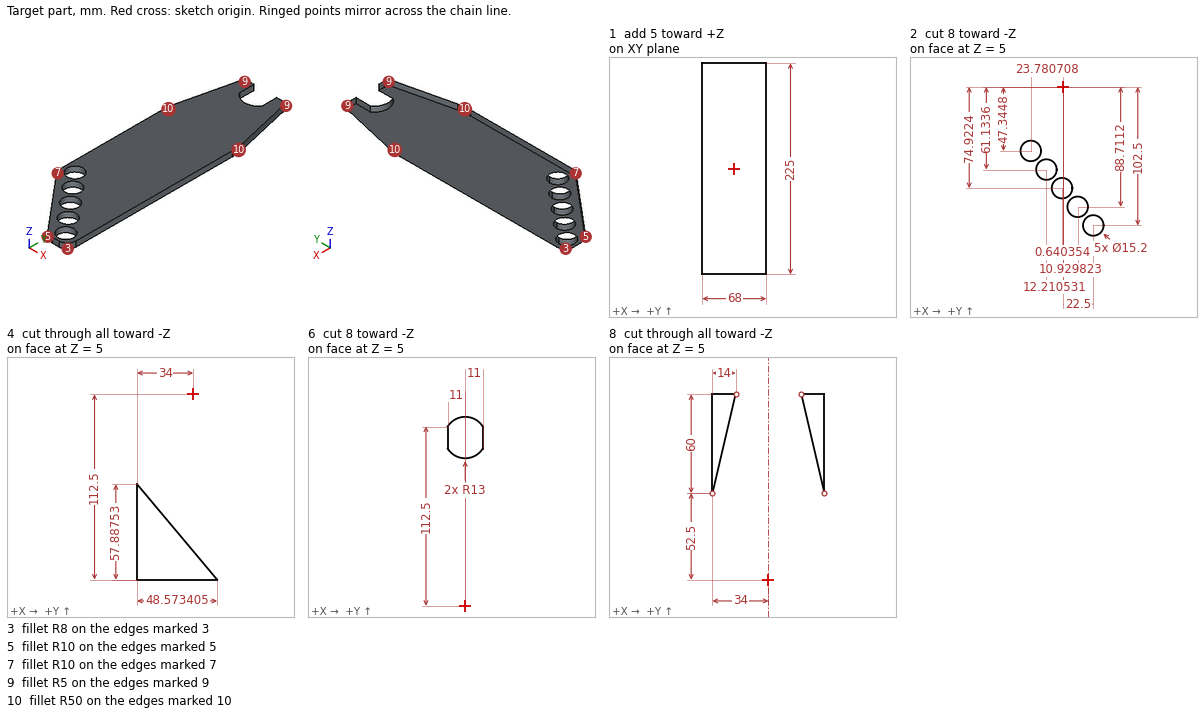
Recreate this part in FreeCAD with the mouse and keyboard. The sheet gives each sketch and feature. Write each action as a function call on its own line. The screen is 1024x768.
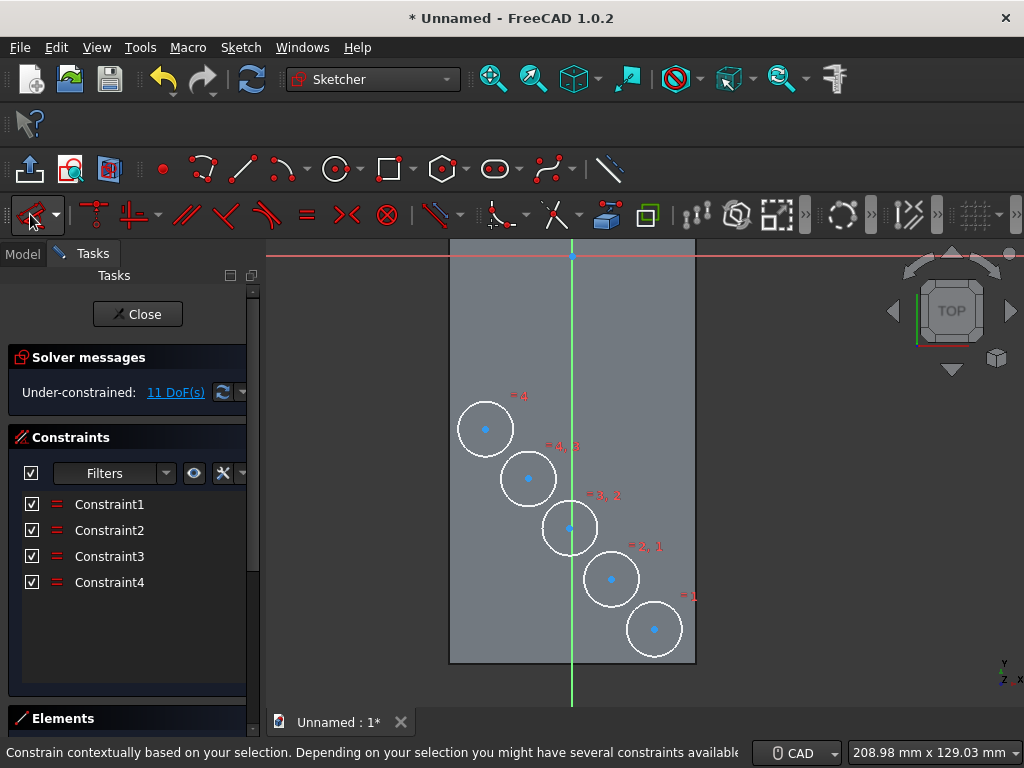
click(674, 610)
click(697, 588)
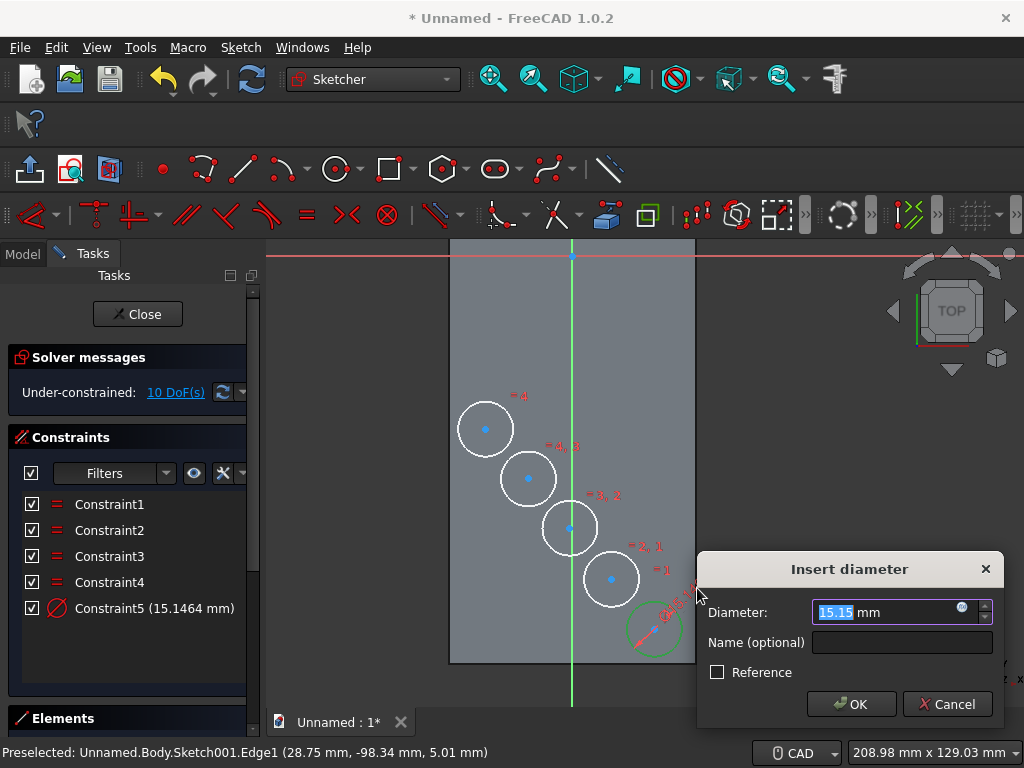
text(15.2)
key(Return)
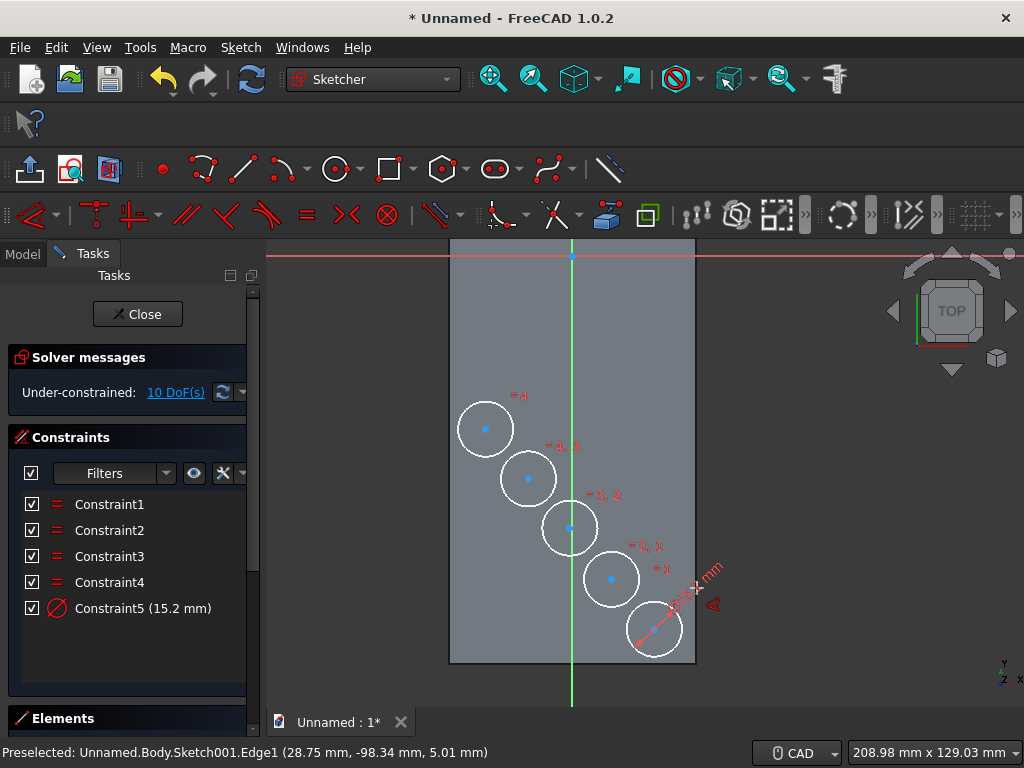
click(654, 629)
click(613, 663)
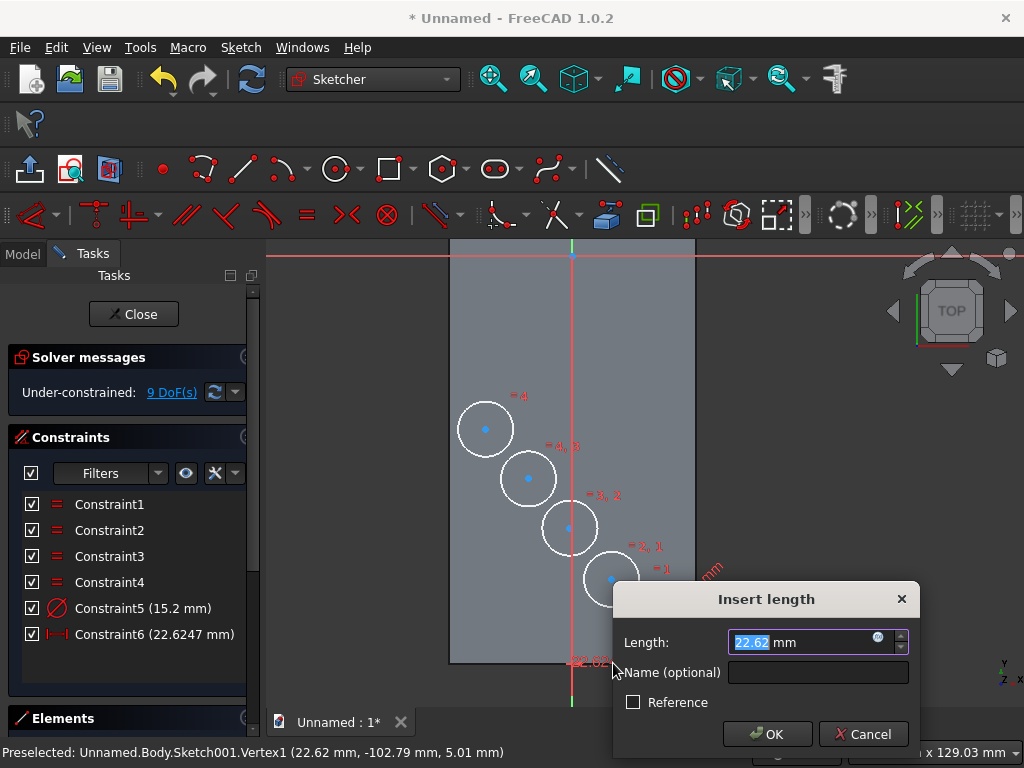
text(22.5)
key(Return)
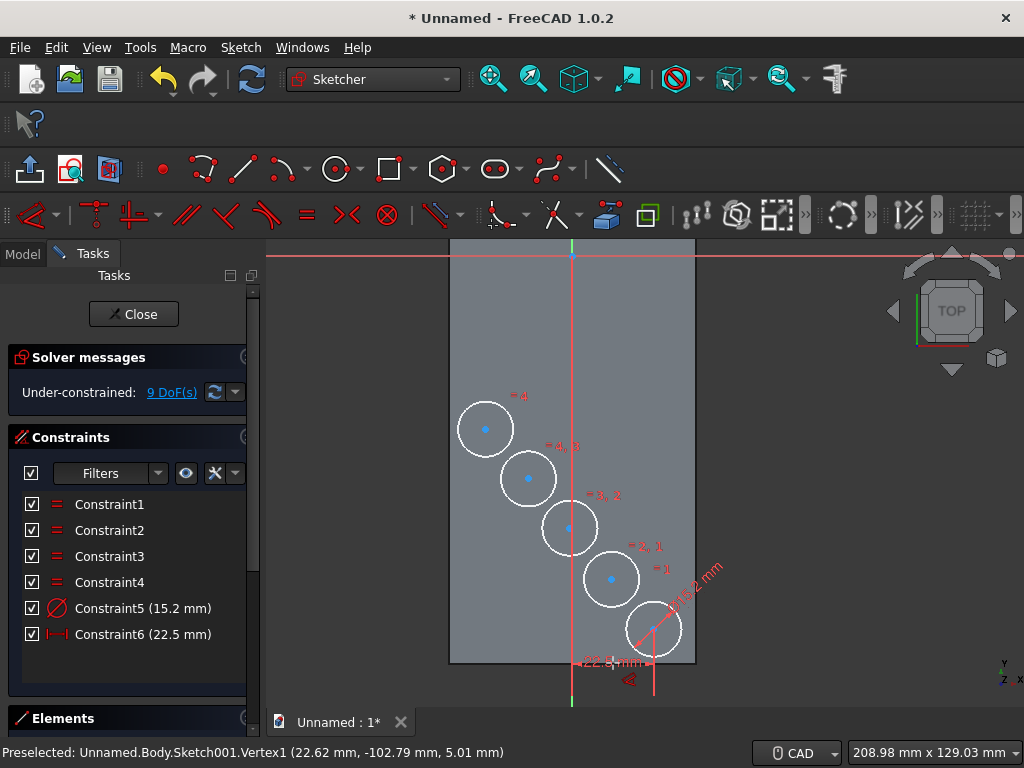
click(654, 629)
click(688, 448)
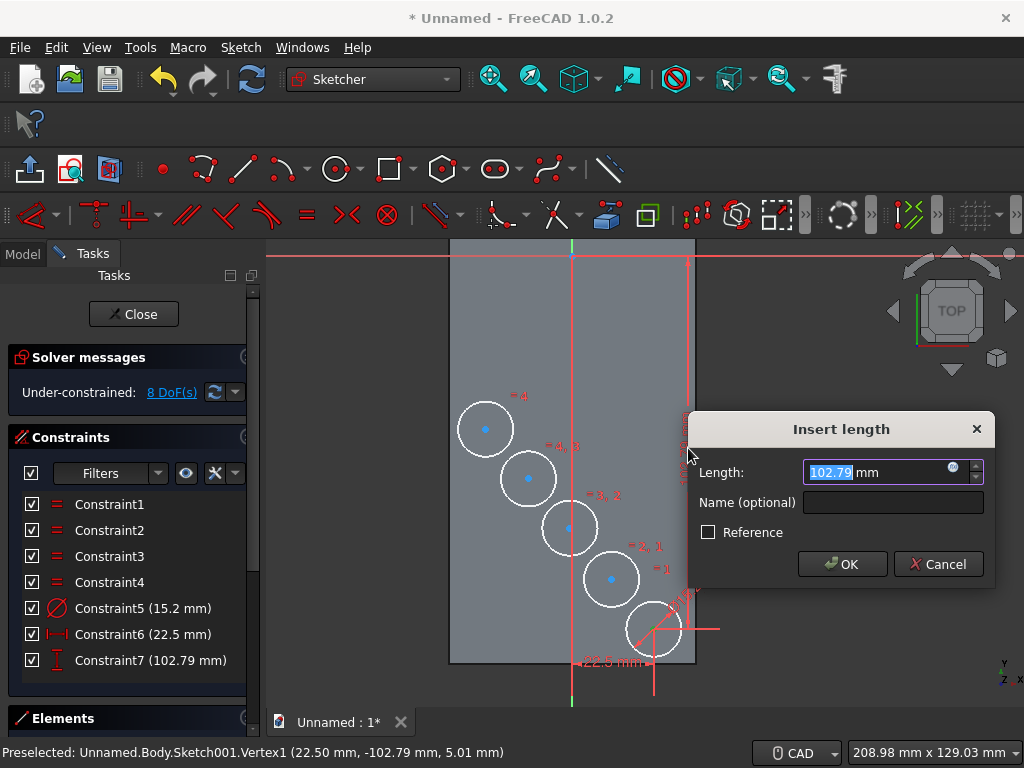
text(102.5)
key(Return)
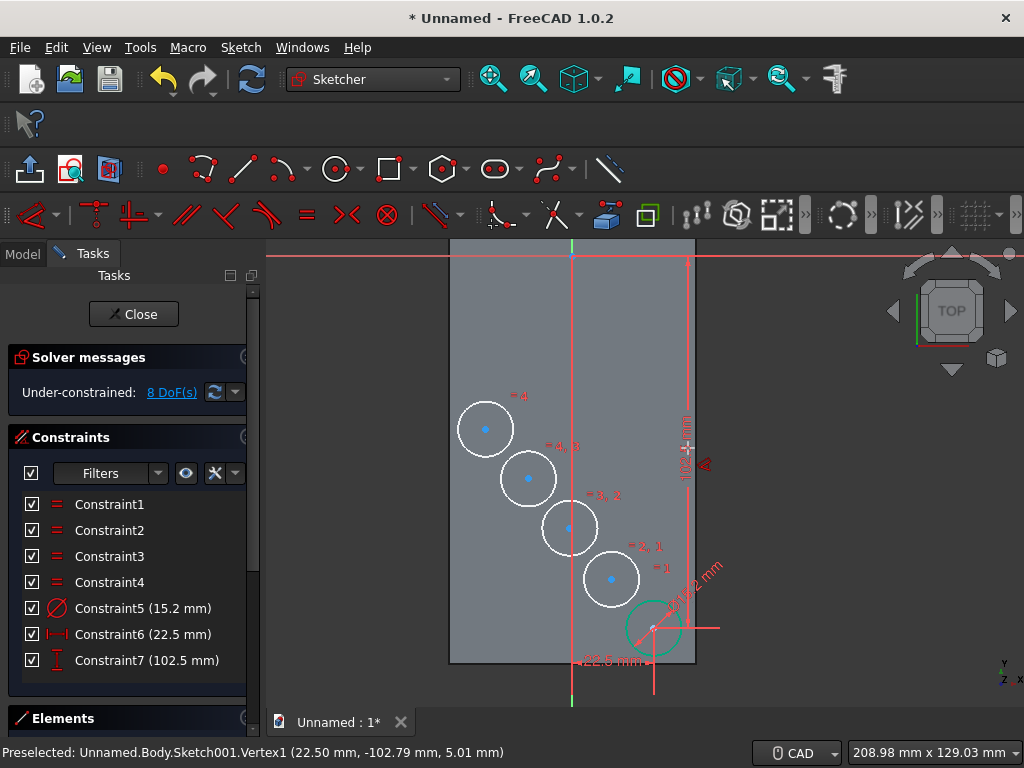
click(612, 579)
click(646, 423)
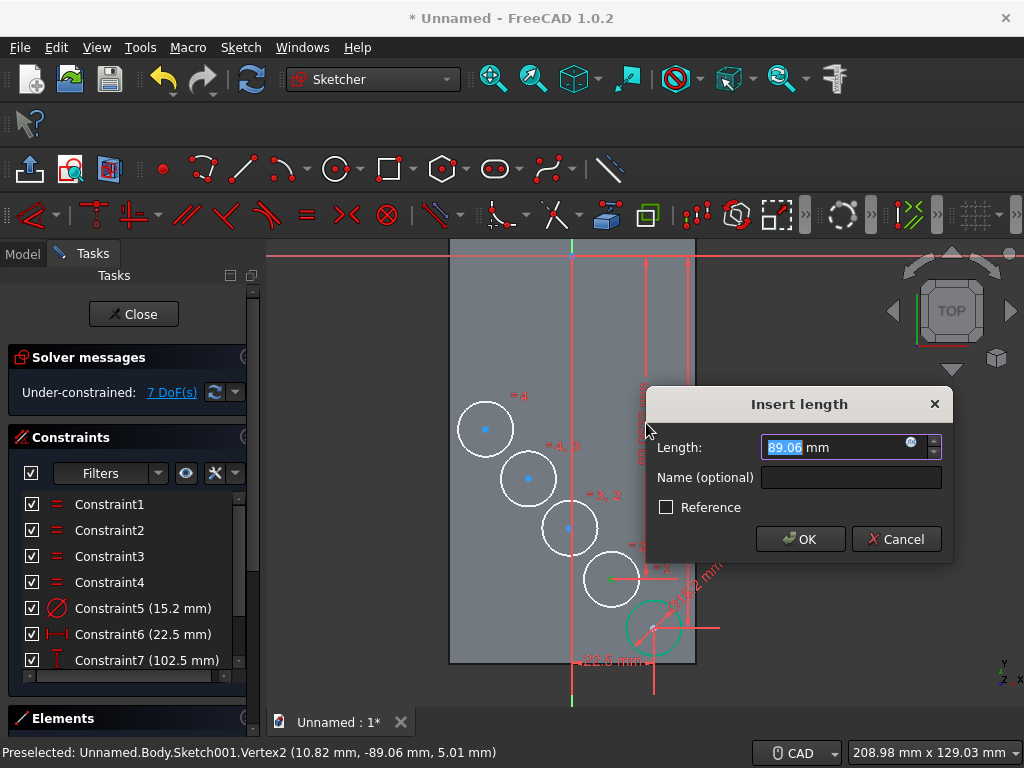
text(88.7112)
key(Return)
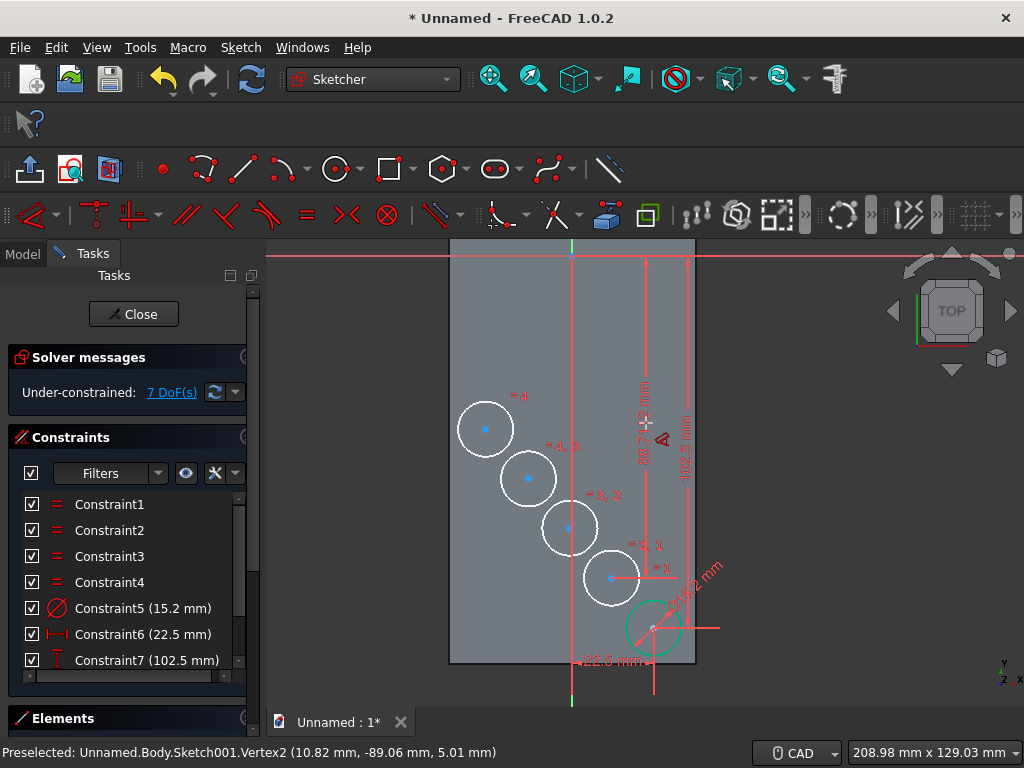
click(570, 528)
click(606, 398)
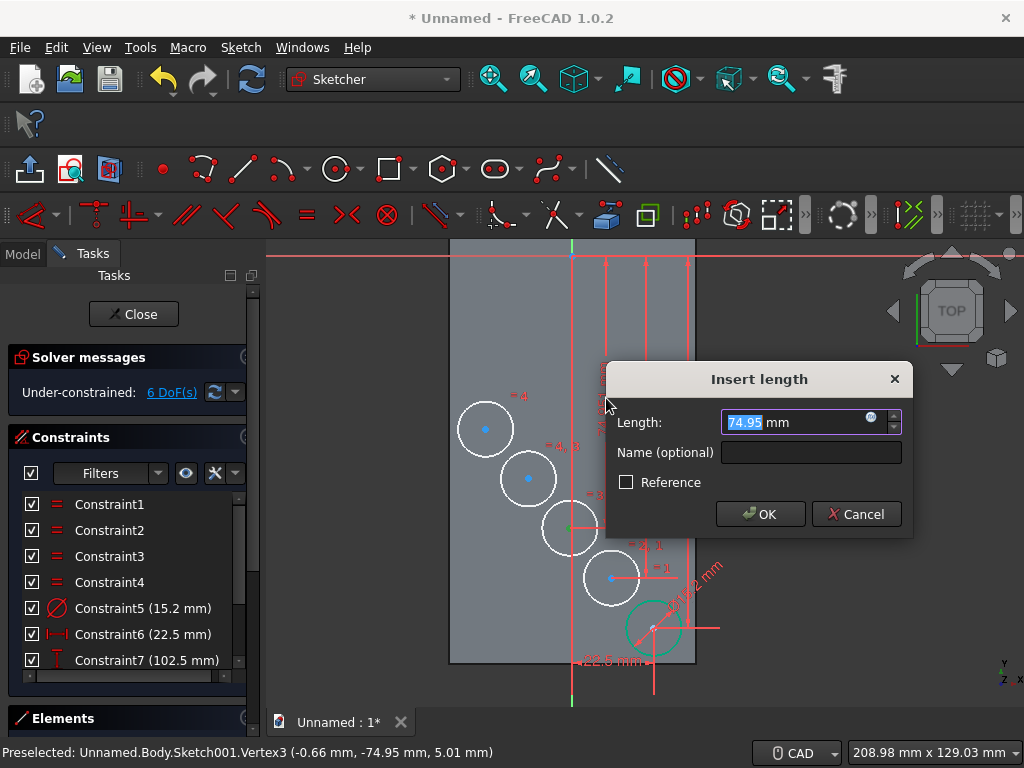
text(74.9224)
key(Return)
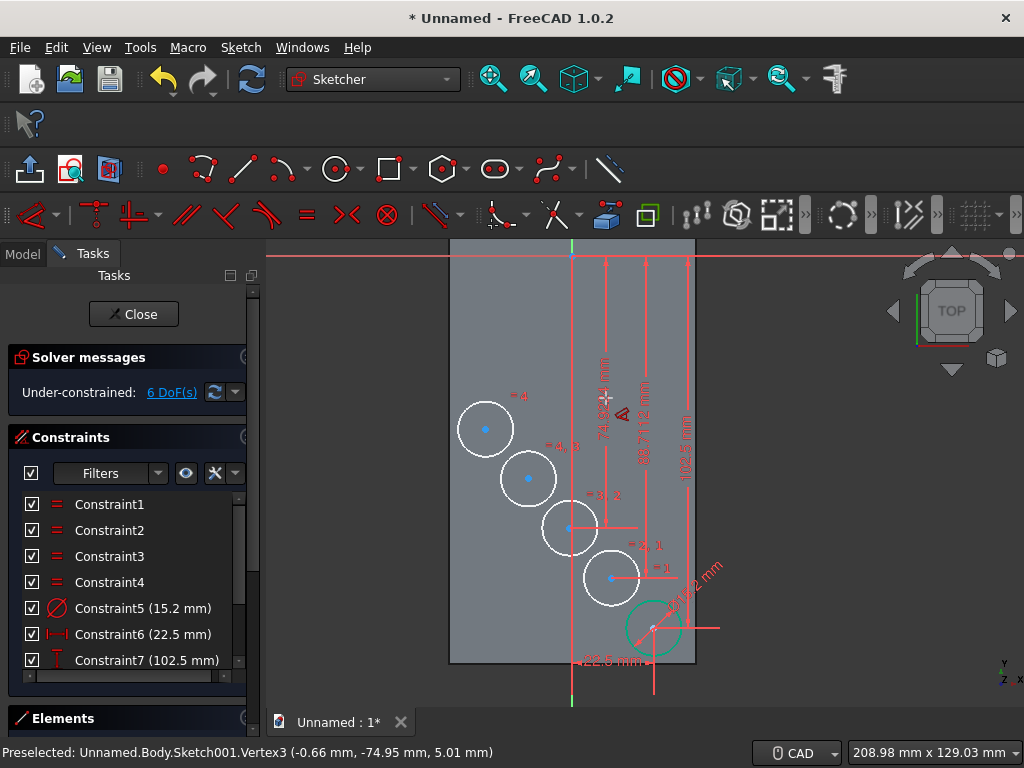
click(528, 479)
click(494, 373)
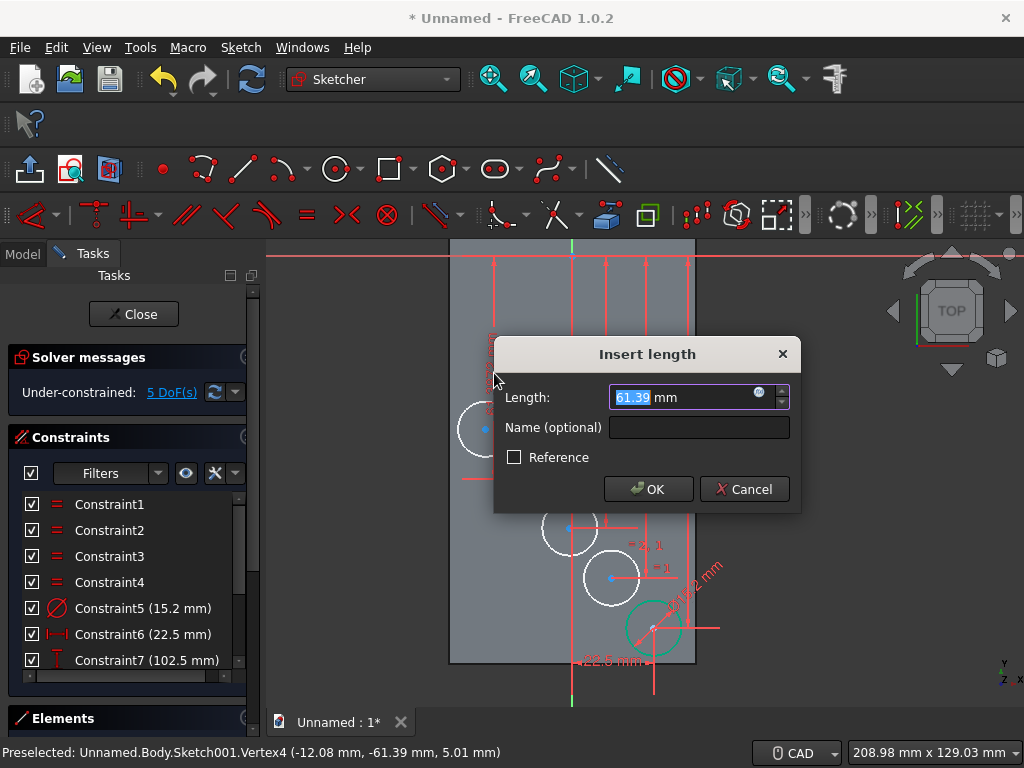
text(61.1336)
key(Return)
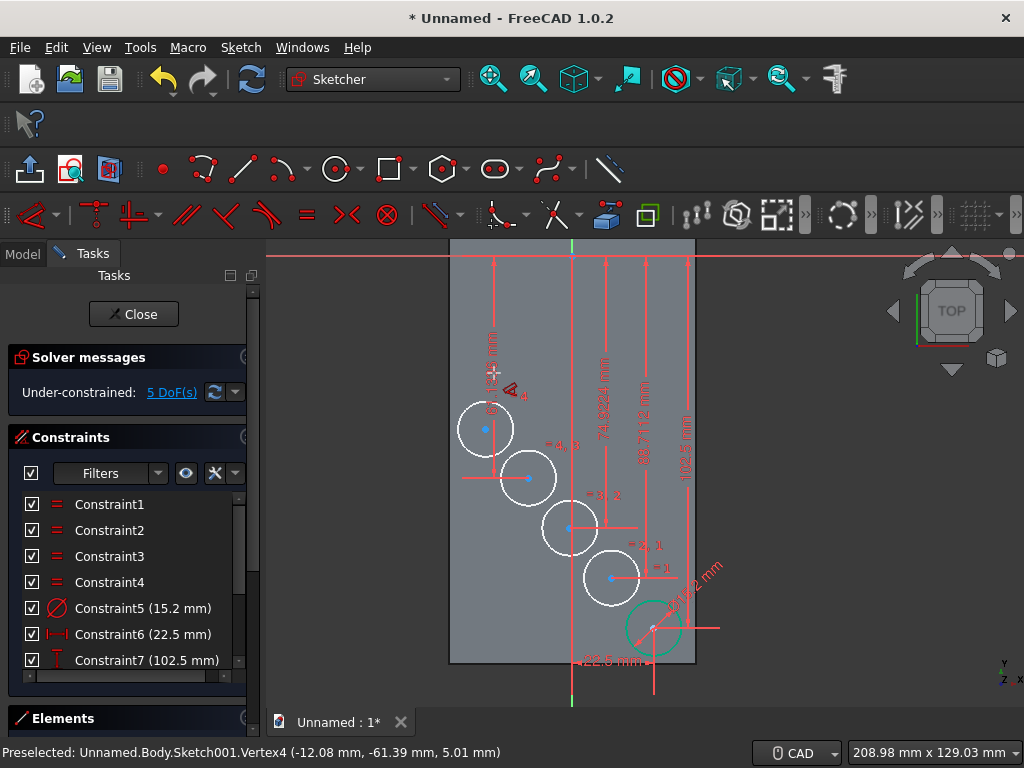
click(486, 429)
click(452, 348)